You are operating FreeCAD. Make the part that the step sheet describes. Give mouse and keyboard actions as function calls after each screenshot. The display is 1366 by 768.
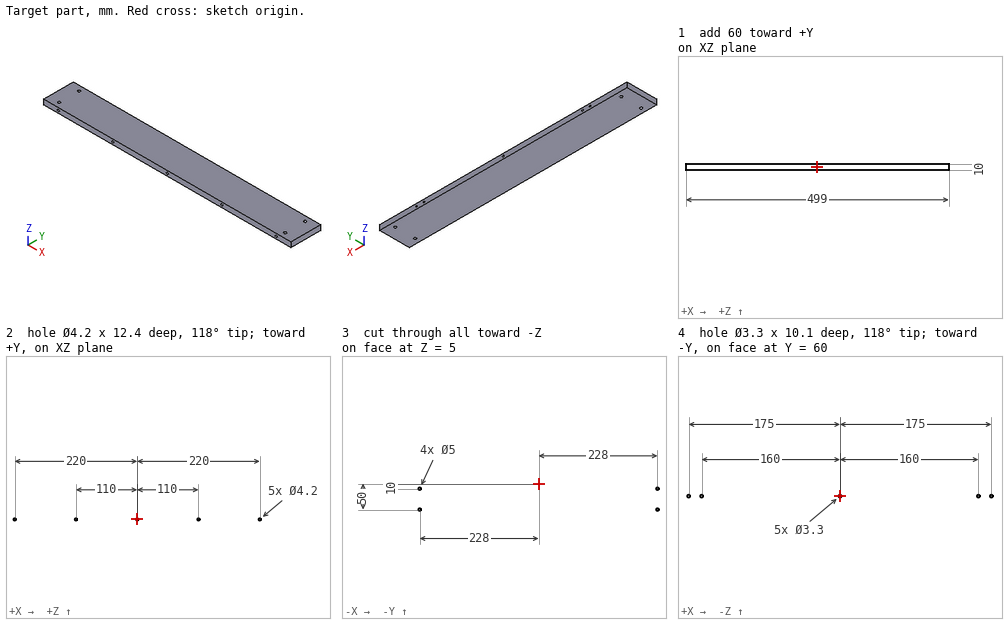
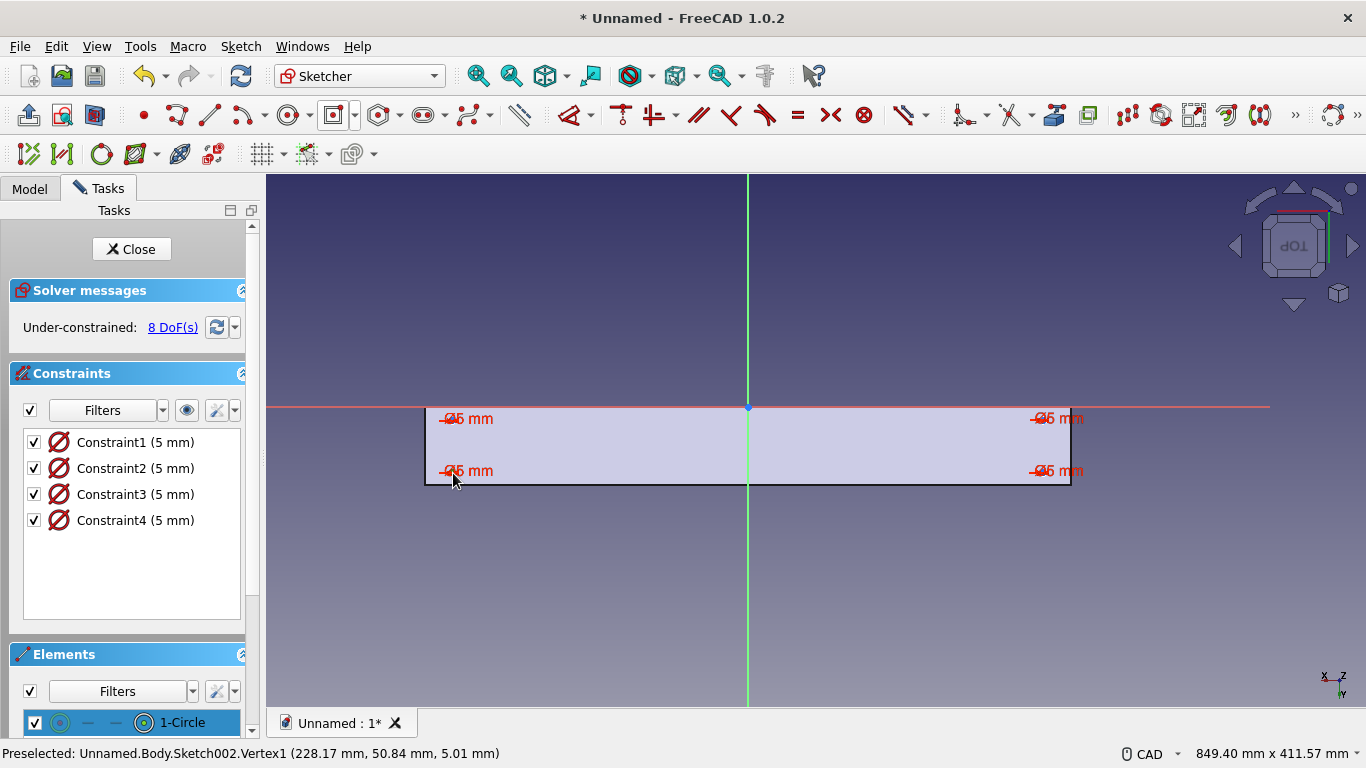
click(453, 421)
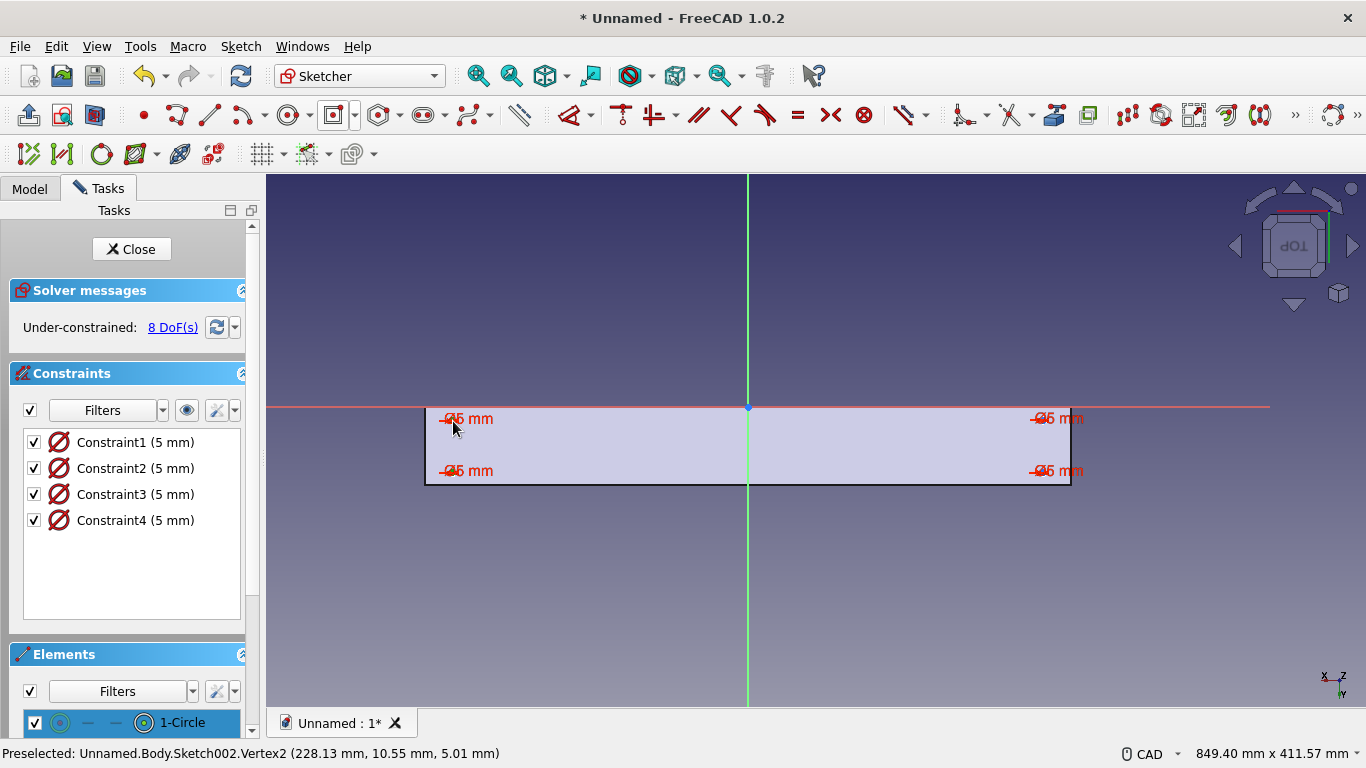
key(v)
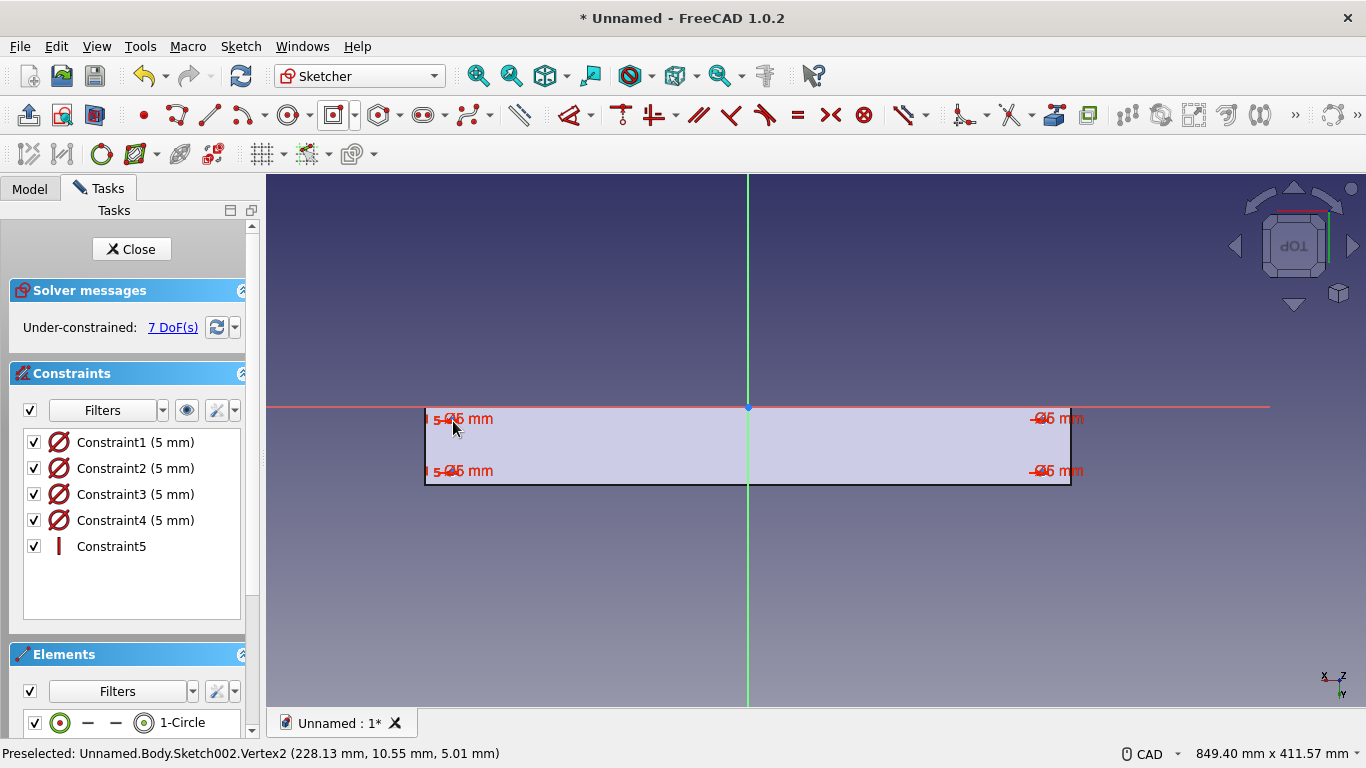
click(453, 421)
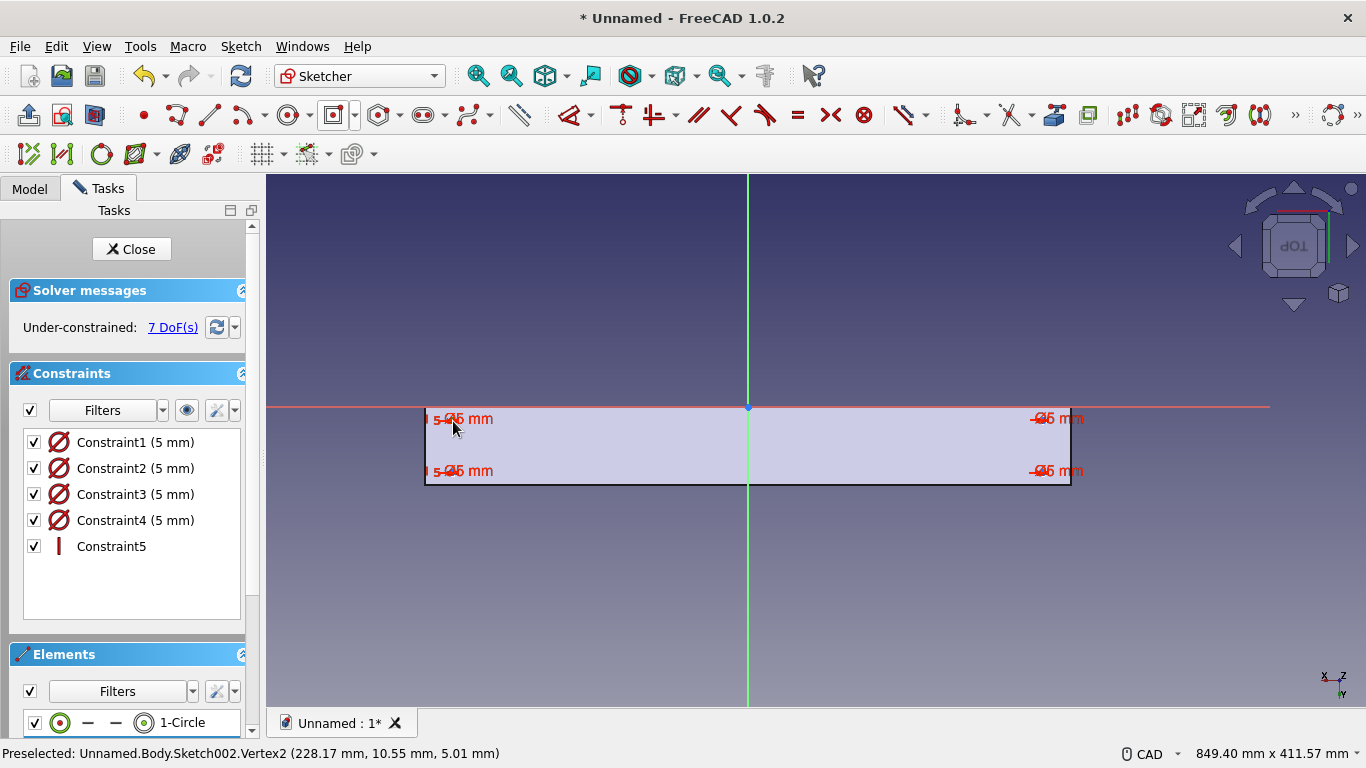
click(1043, 420)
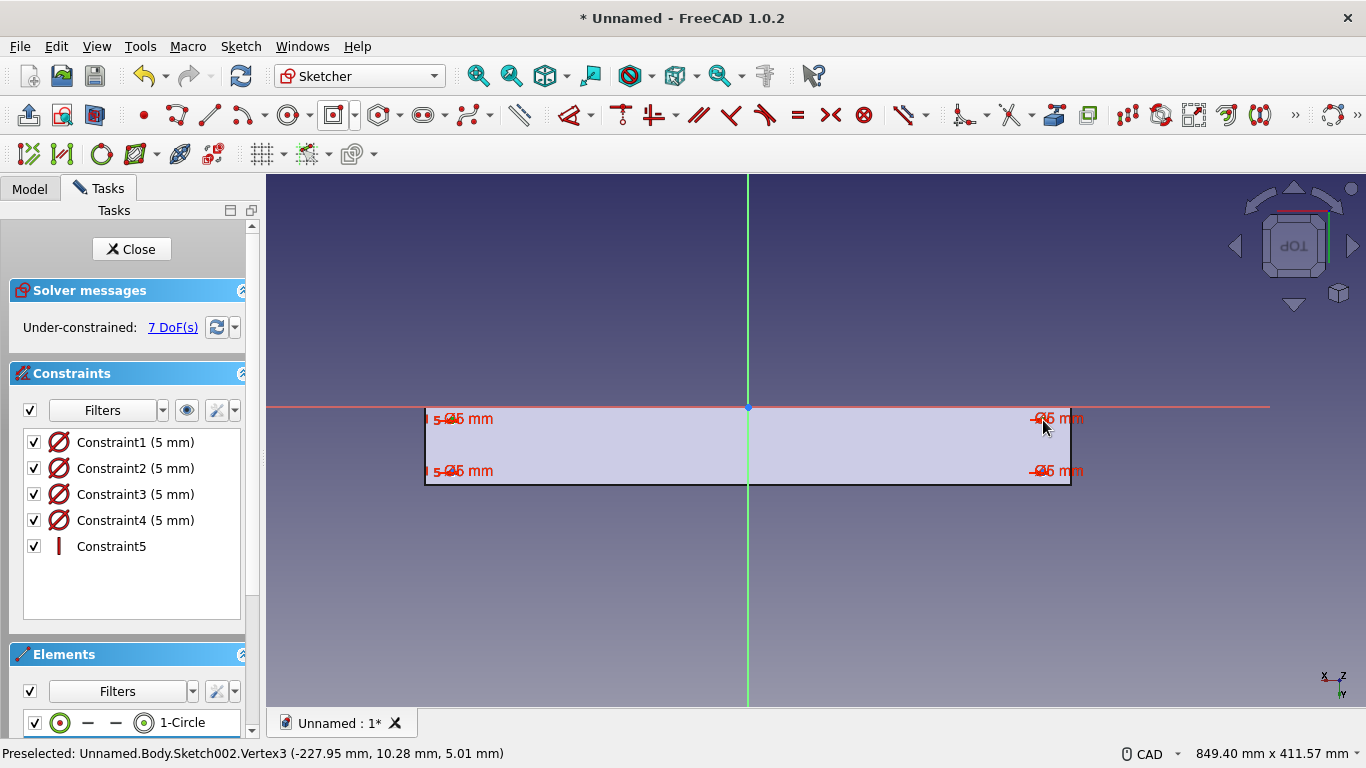
key(h)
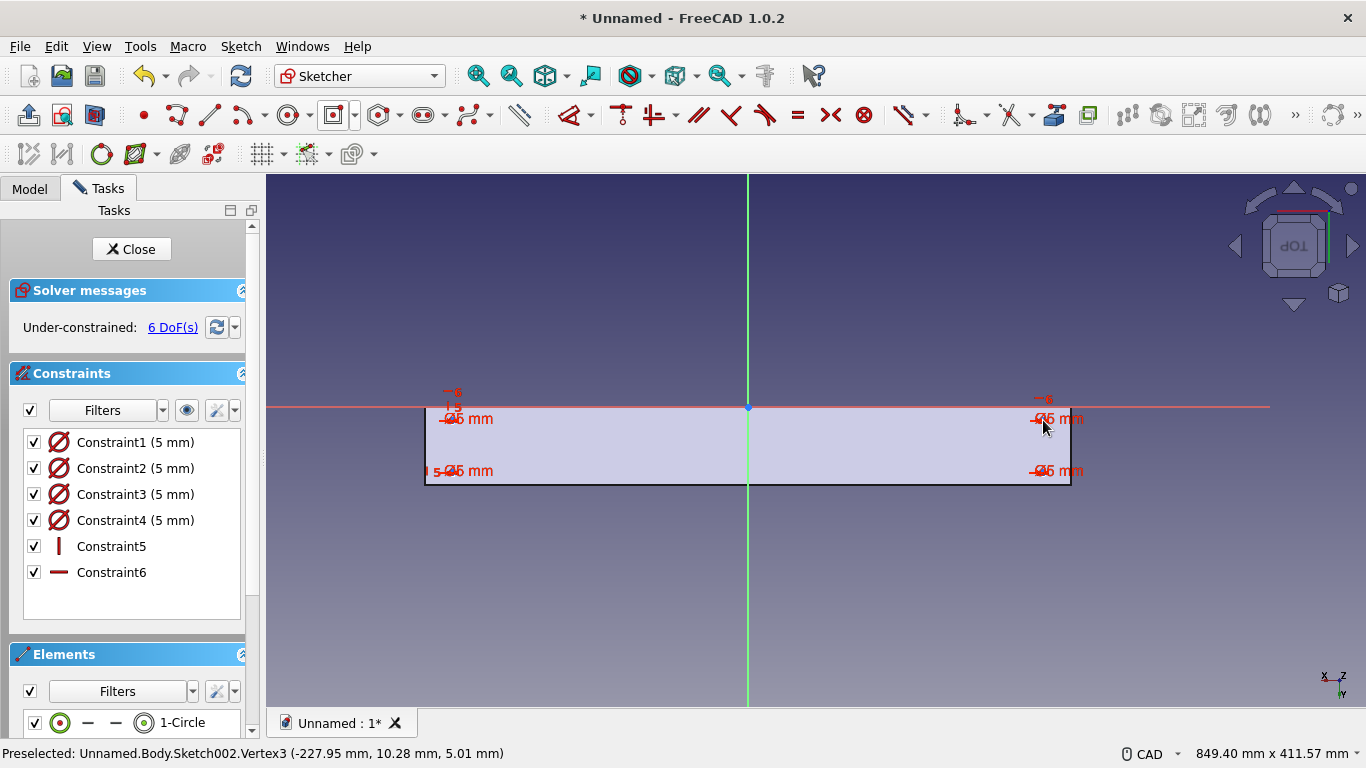
click(1043, 421)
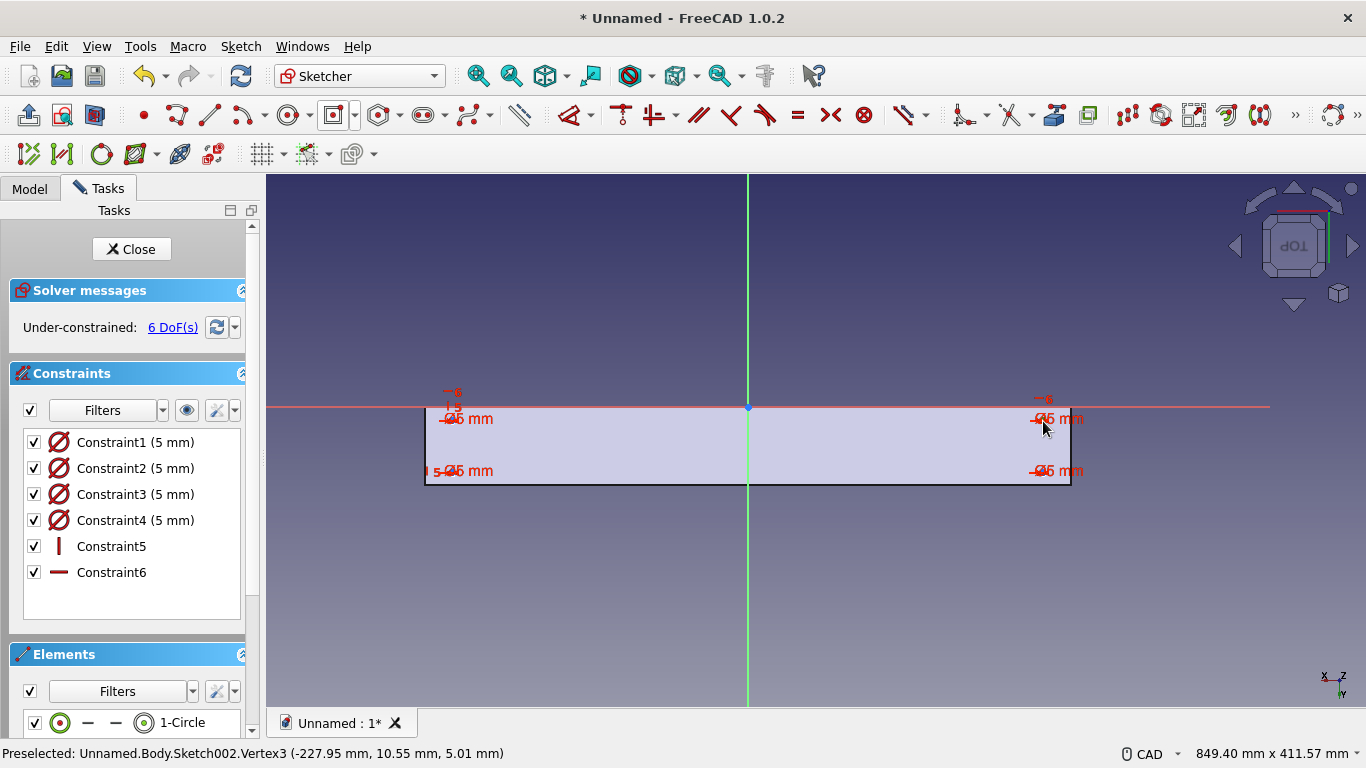
click(1043, 473)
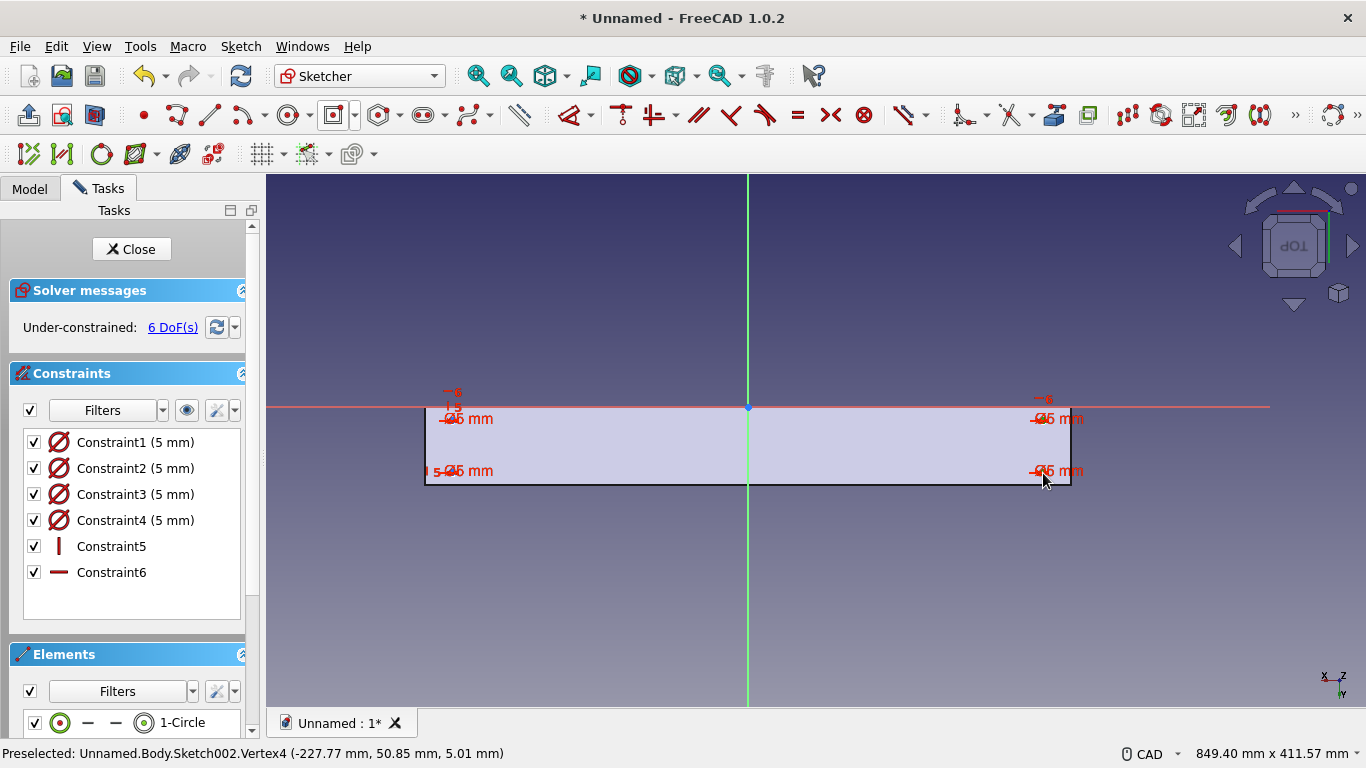
key(v)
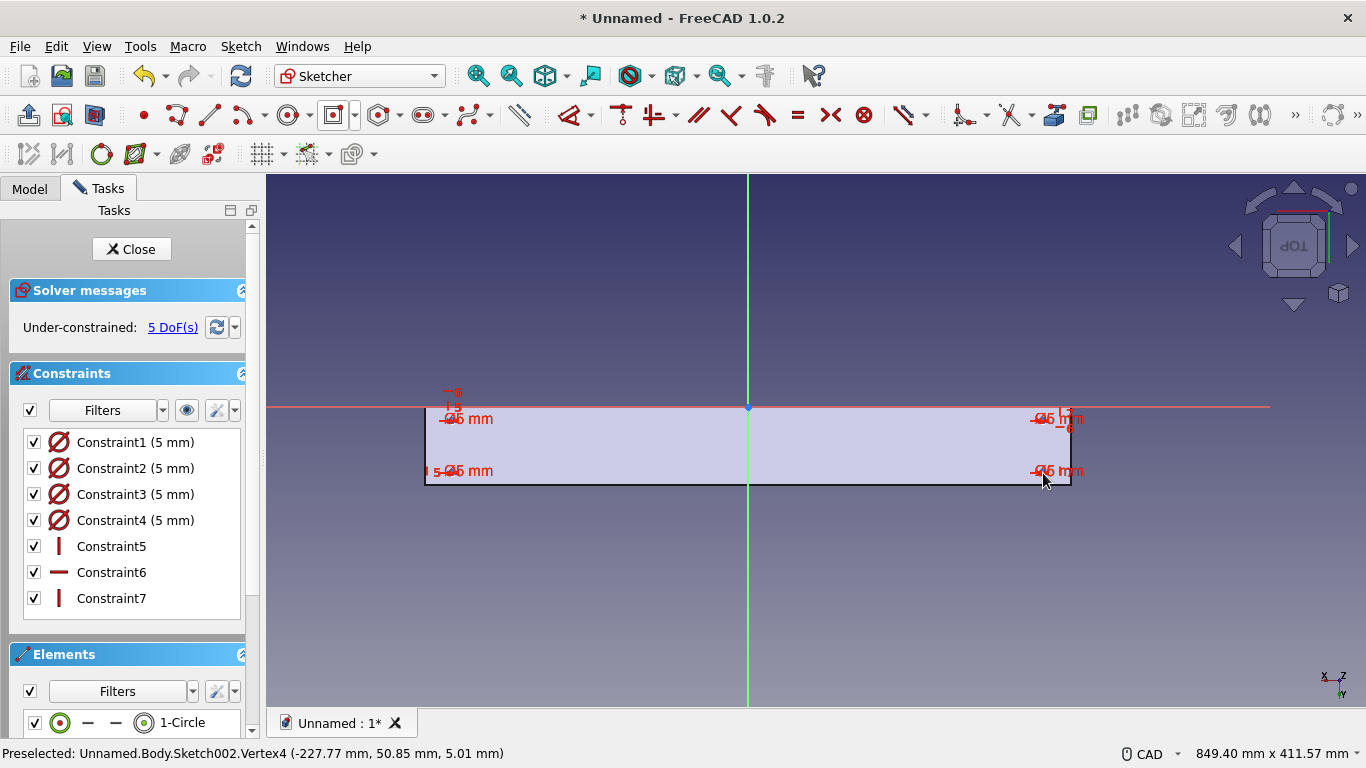
click(453, 473)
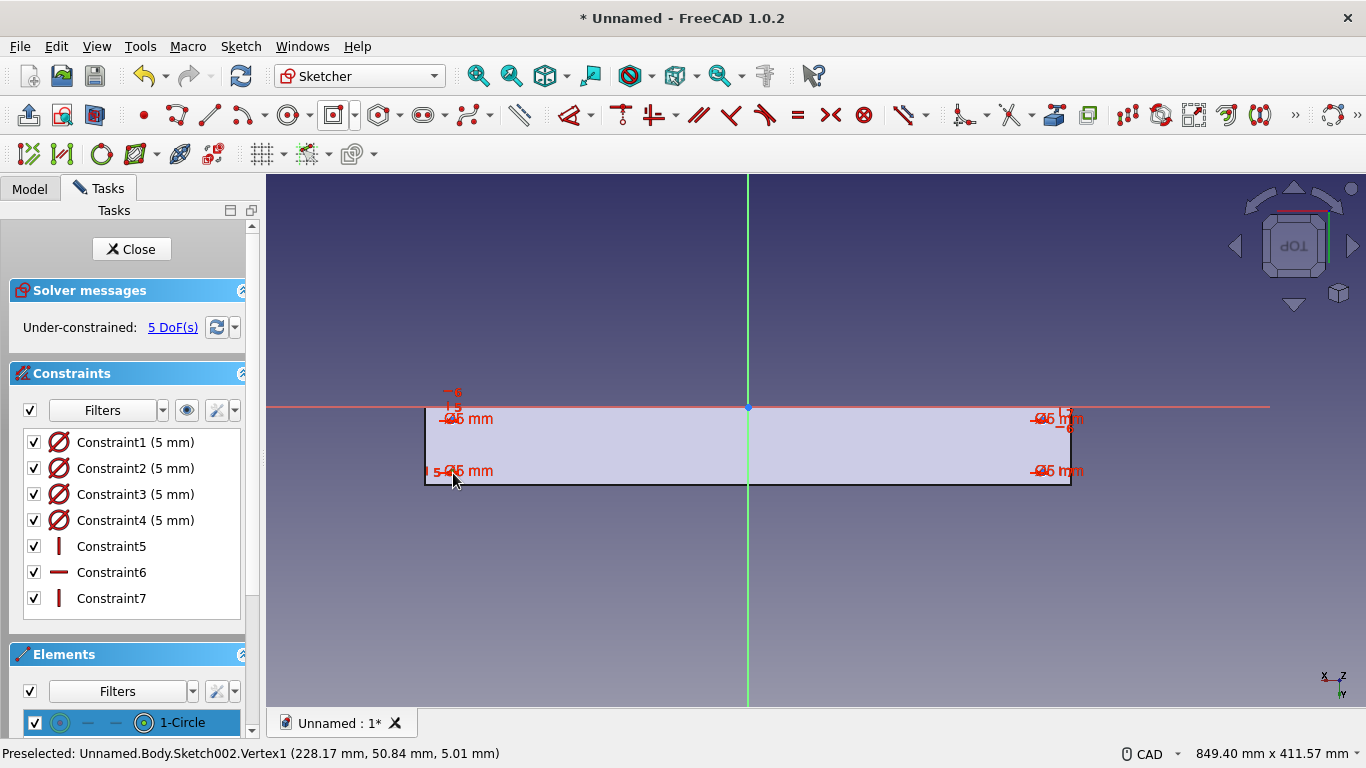
click(1043, 473)